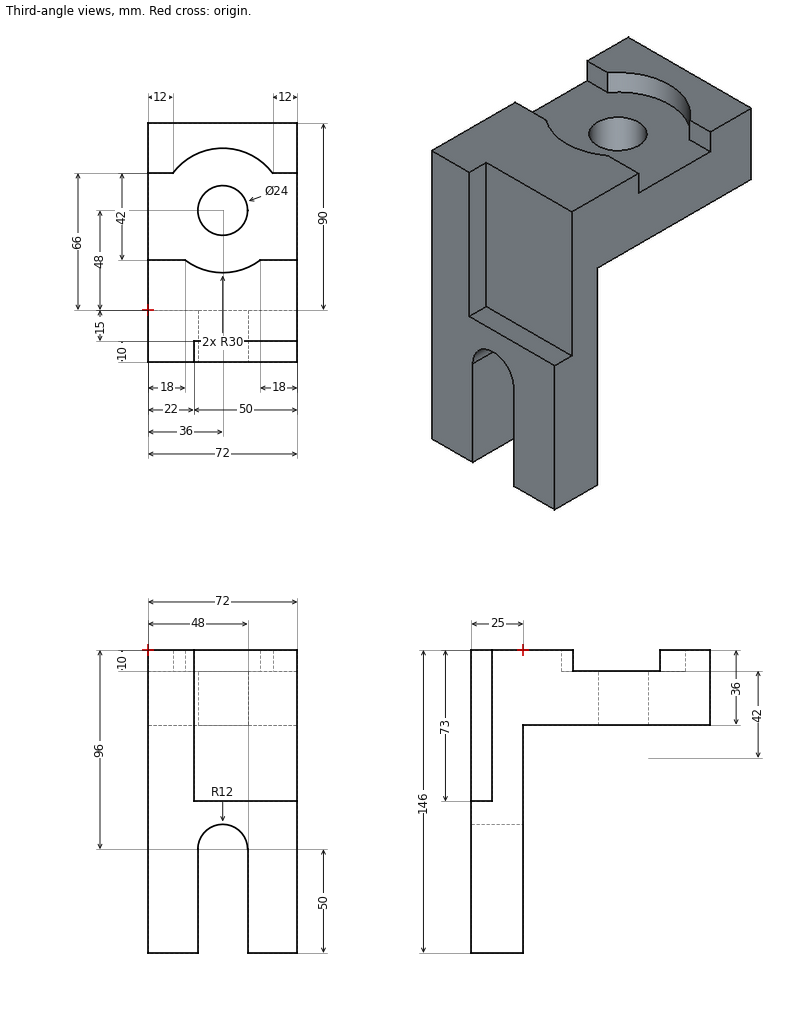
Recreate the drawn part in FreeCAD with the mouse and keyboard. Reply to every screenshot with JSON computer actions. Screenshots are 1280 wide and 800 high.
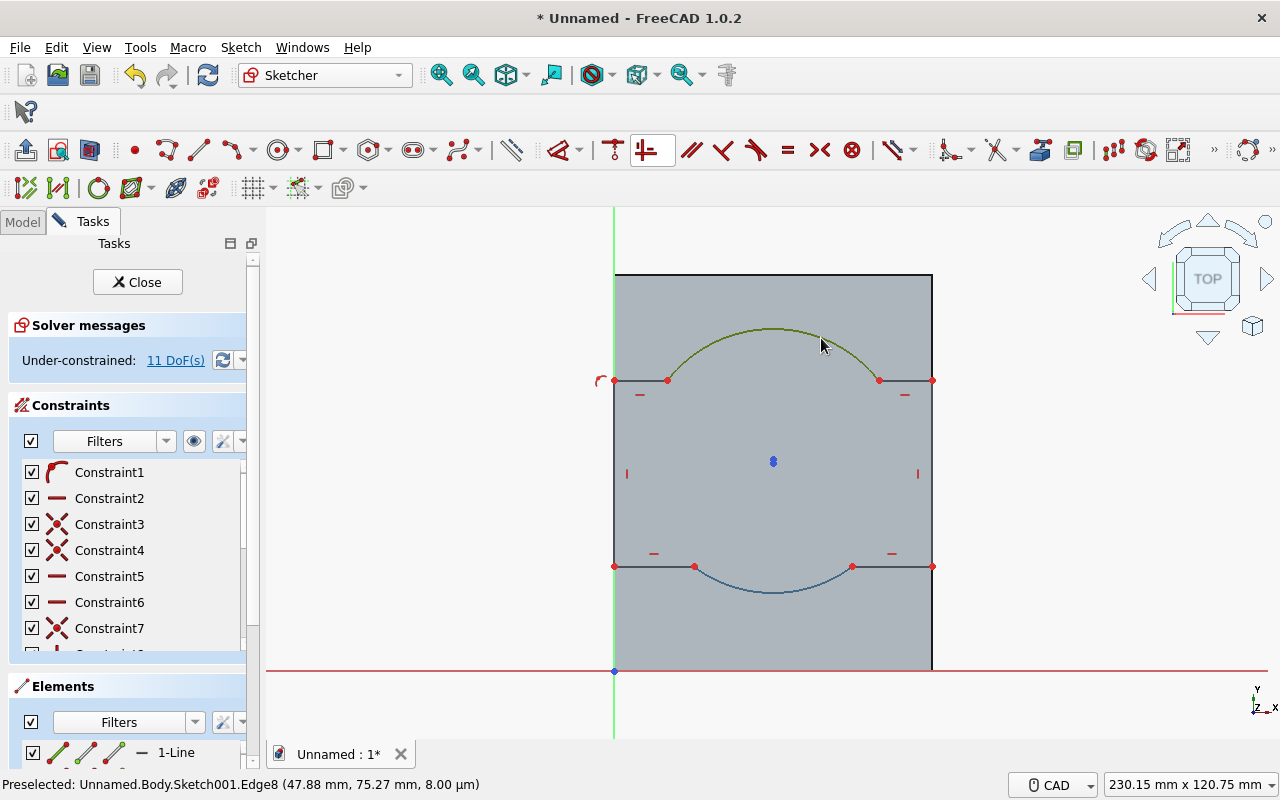
{"action": "left_click", "coordinate": [614, 150]}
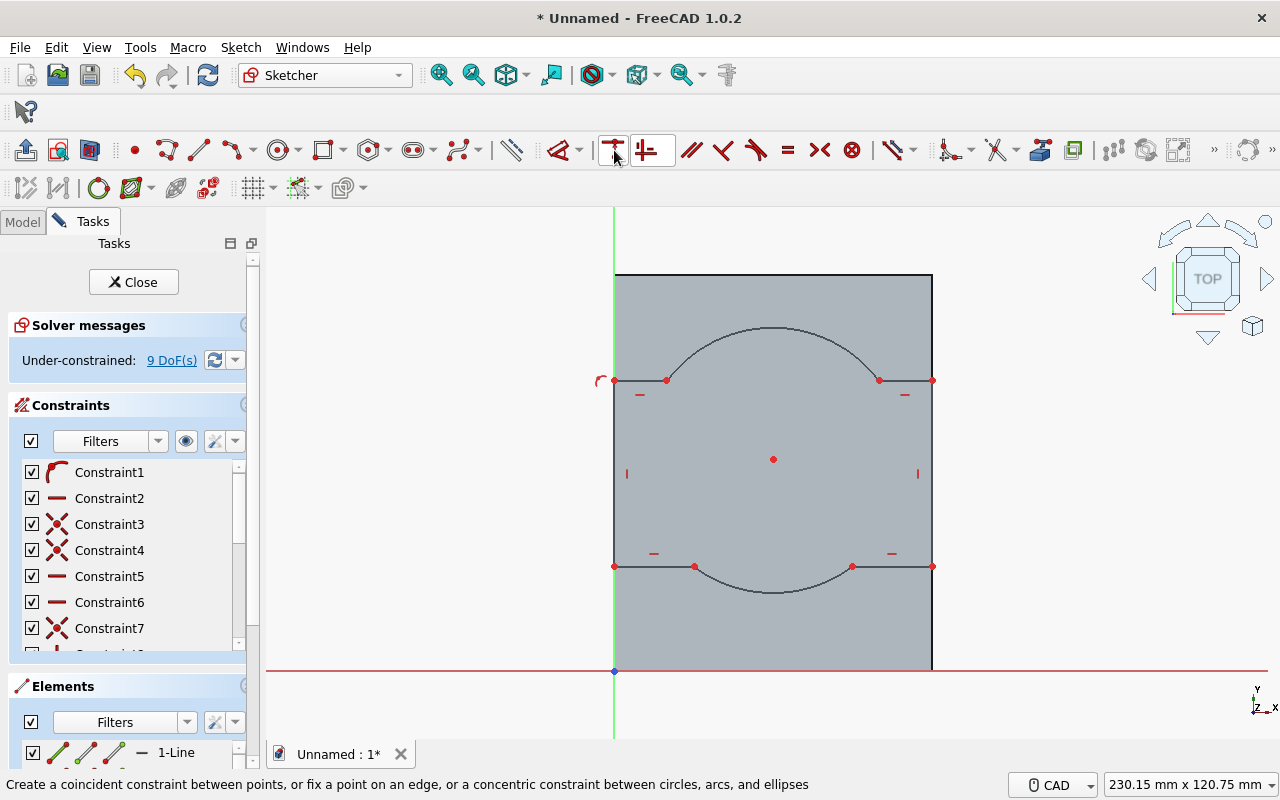
{"action": "left_click", "coordinate": [740, 589]}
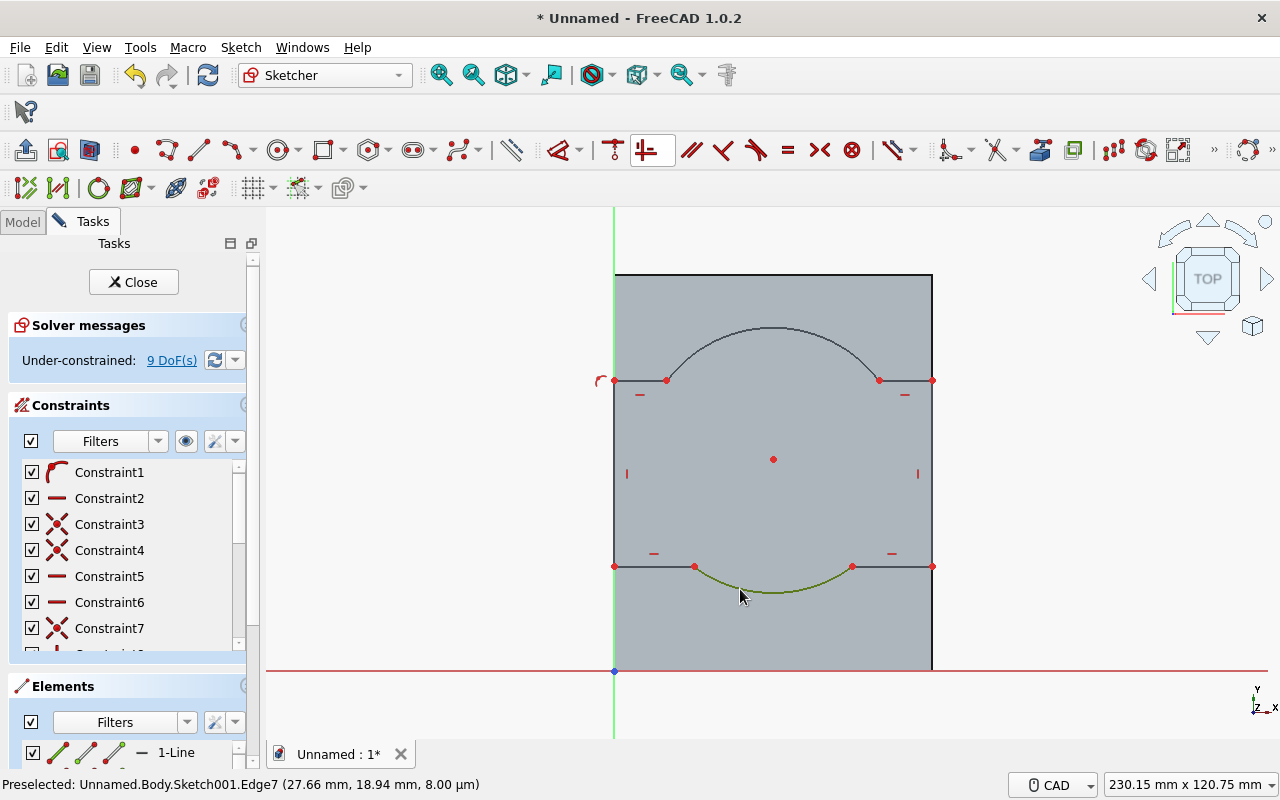
{"action": "left_click", "coordinate": [821, 337]}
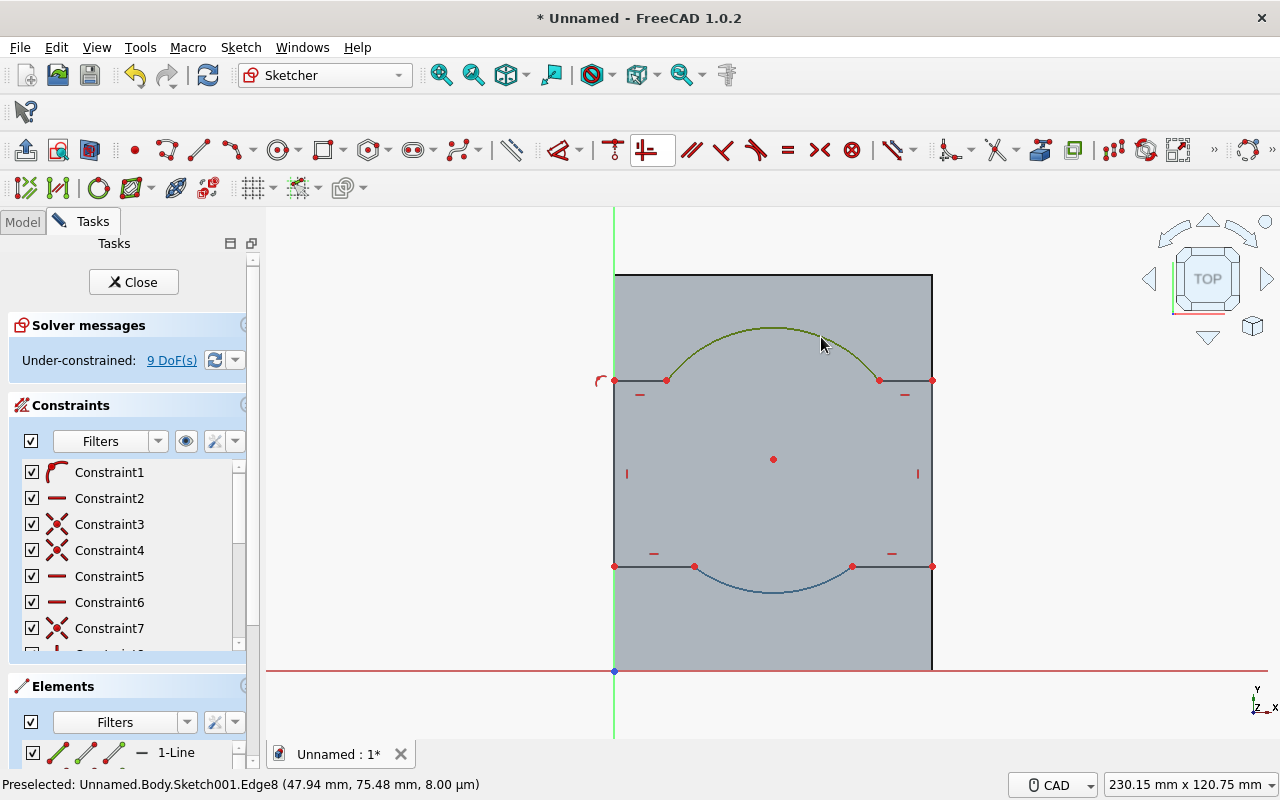
{"action": "left_click", "coordinate": [788, 150]}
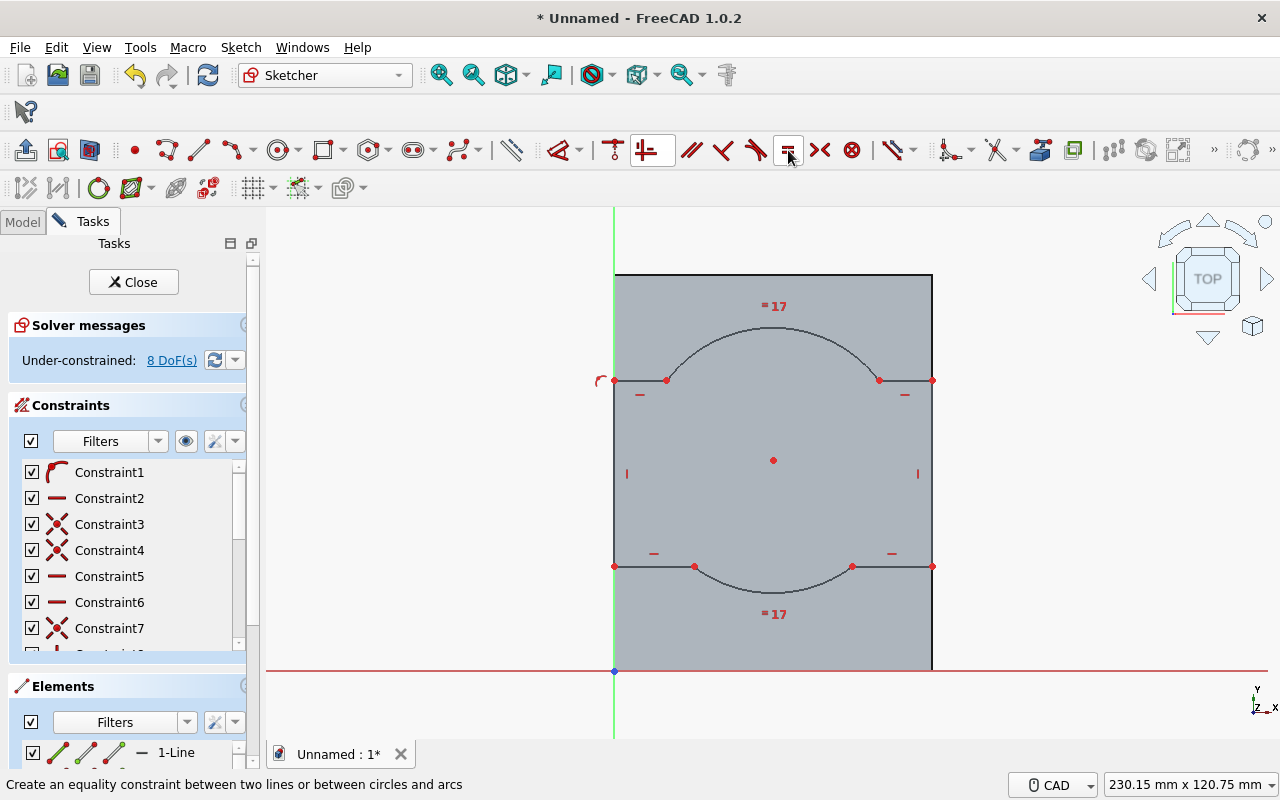
{"action": "left_click", "coordinate": [558, 150]}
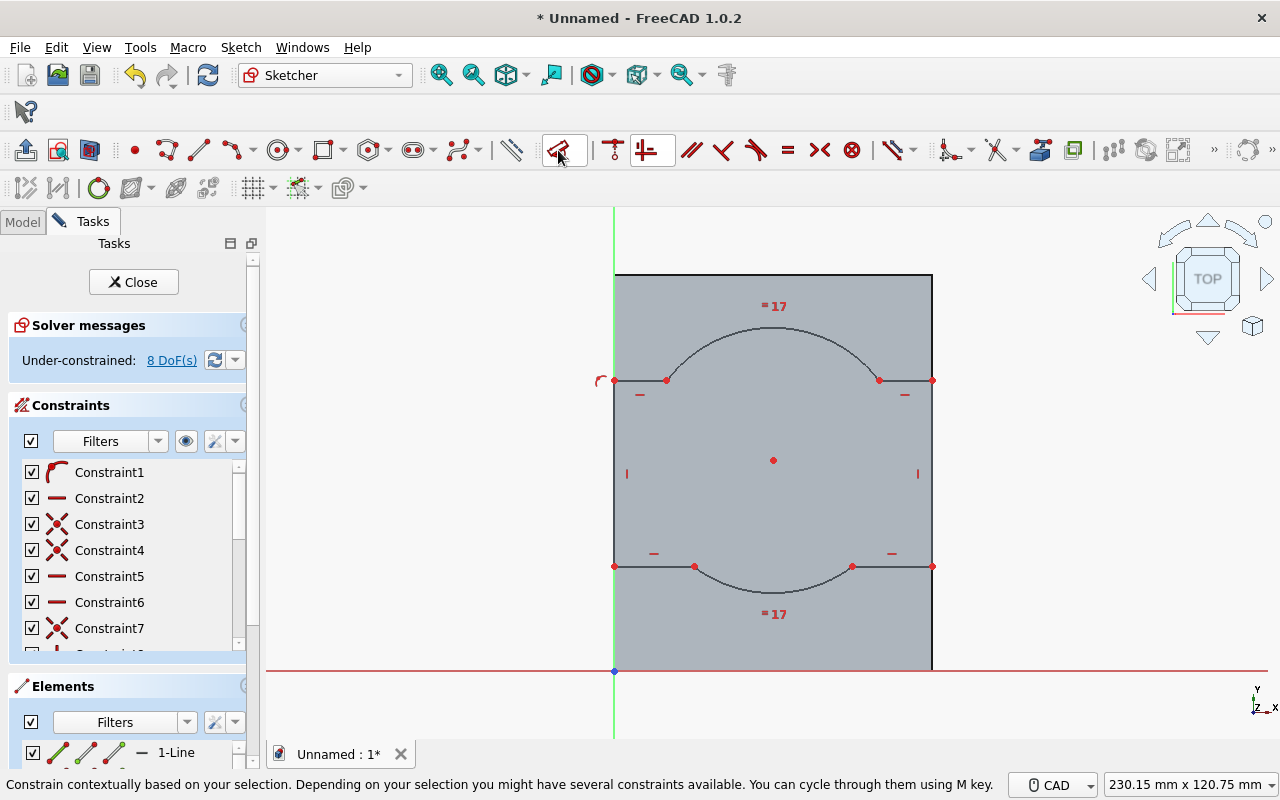
{"action": "left_click", "coordinate": [740, 589]}
{"action": "left_click", "coordinate": [732, 620]}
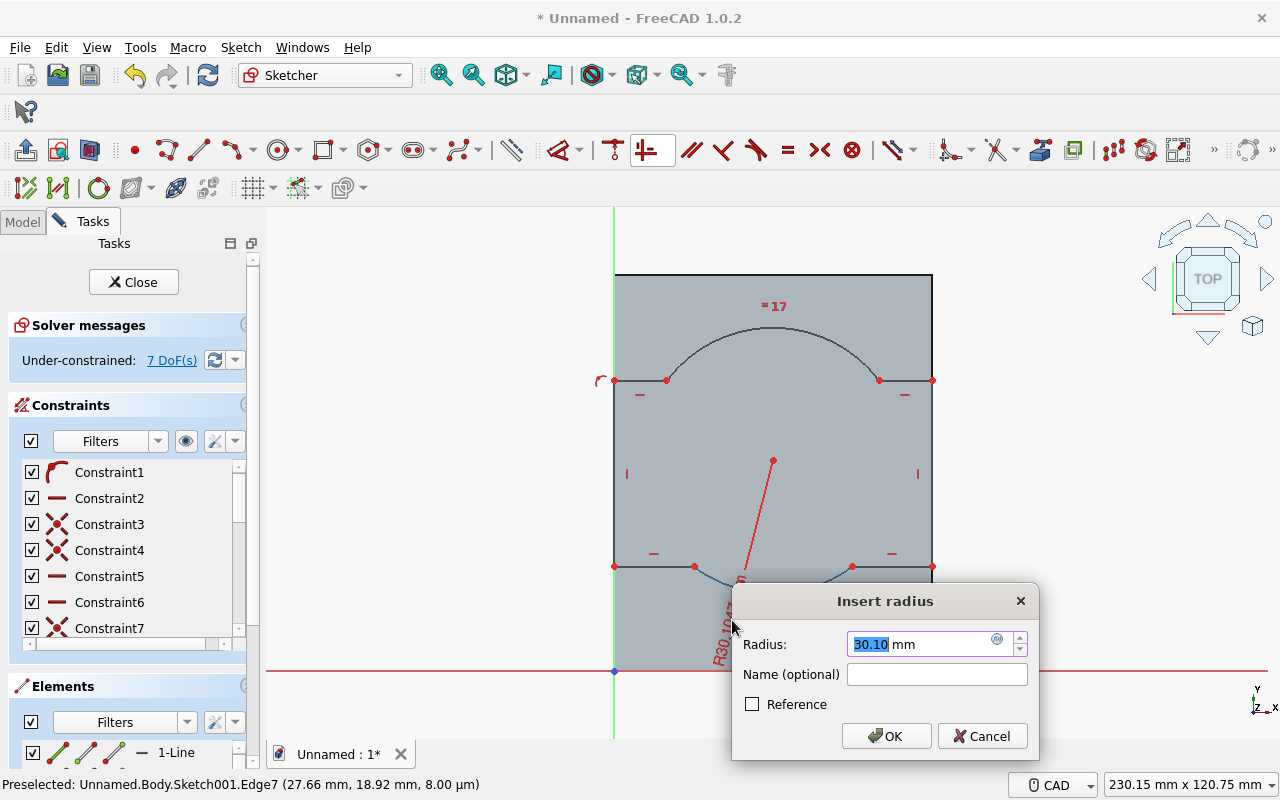
{"action": "type", "text": "30"}
{"action": "key", "text": "Return"}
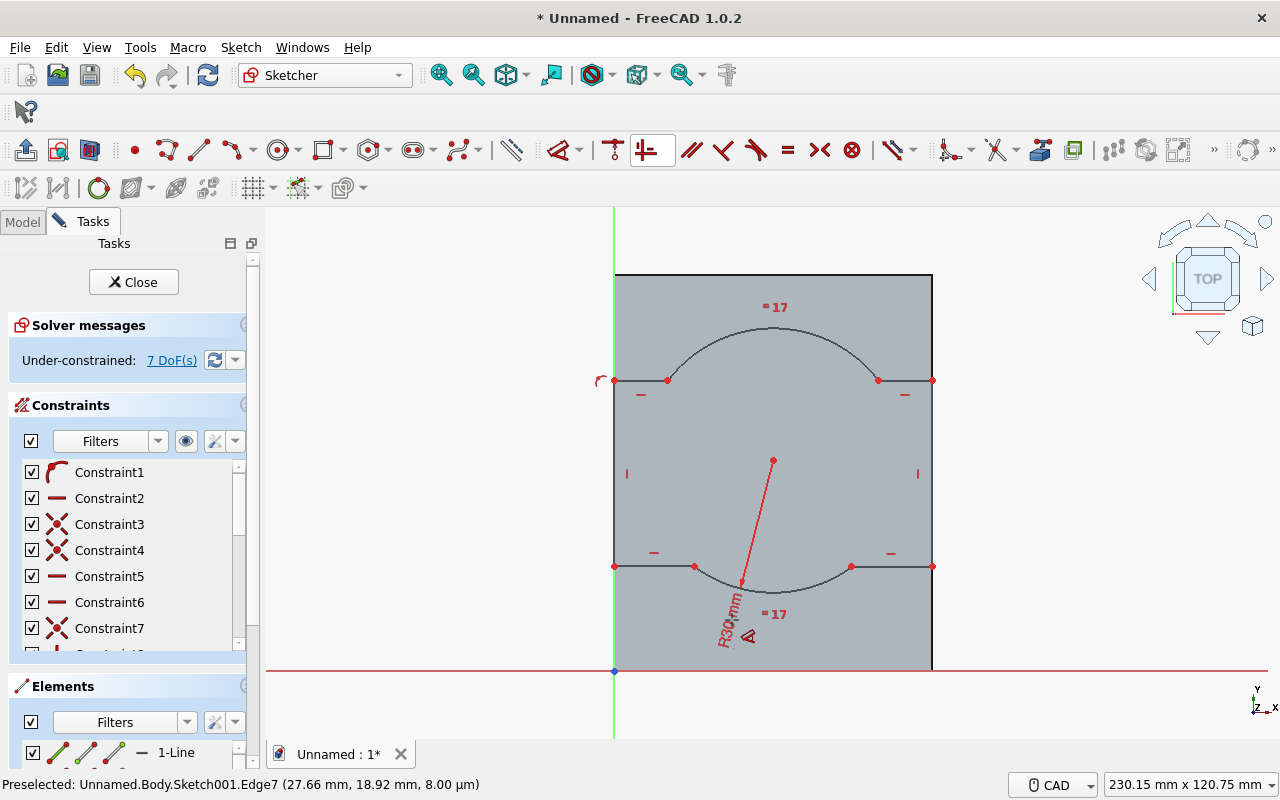
{"action": "left_click", "coordinate": [652, 381]}
{"action": "left_click", "coordinate": [641, 347]}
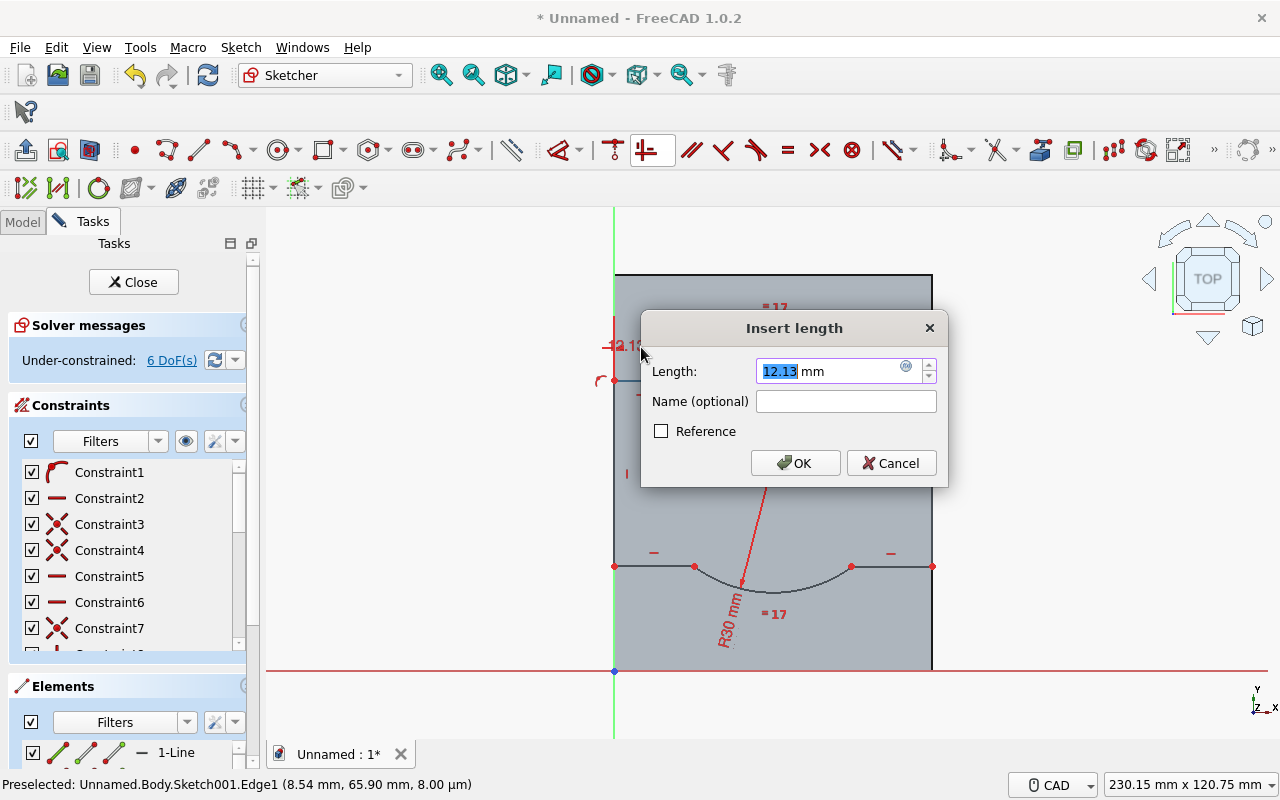
{"action": "type", "text": "12"}
{"action": "key", "text": "Return"}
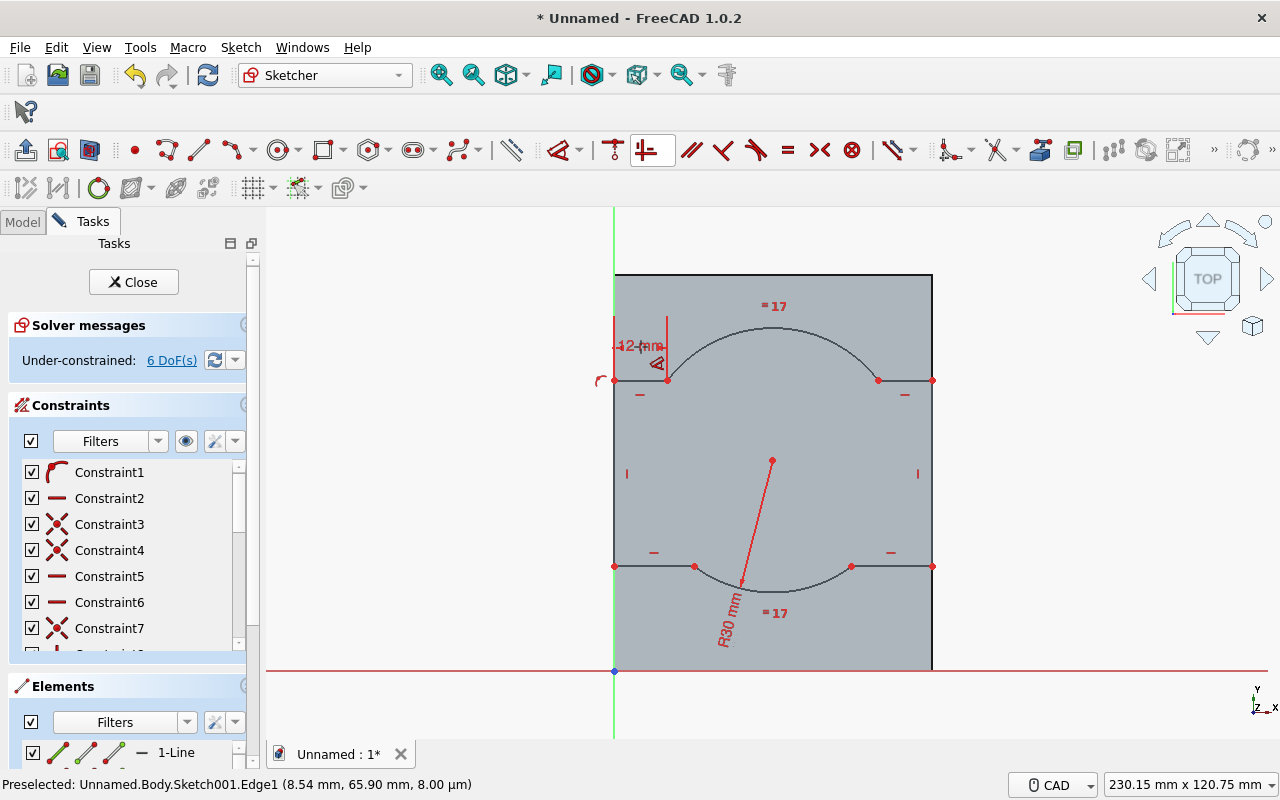
{"action": "left_click", "coordinate": [614, 437]}
{"action": "left_click", "coordinate": [580, 474]}